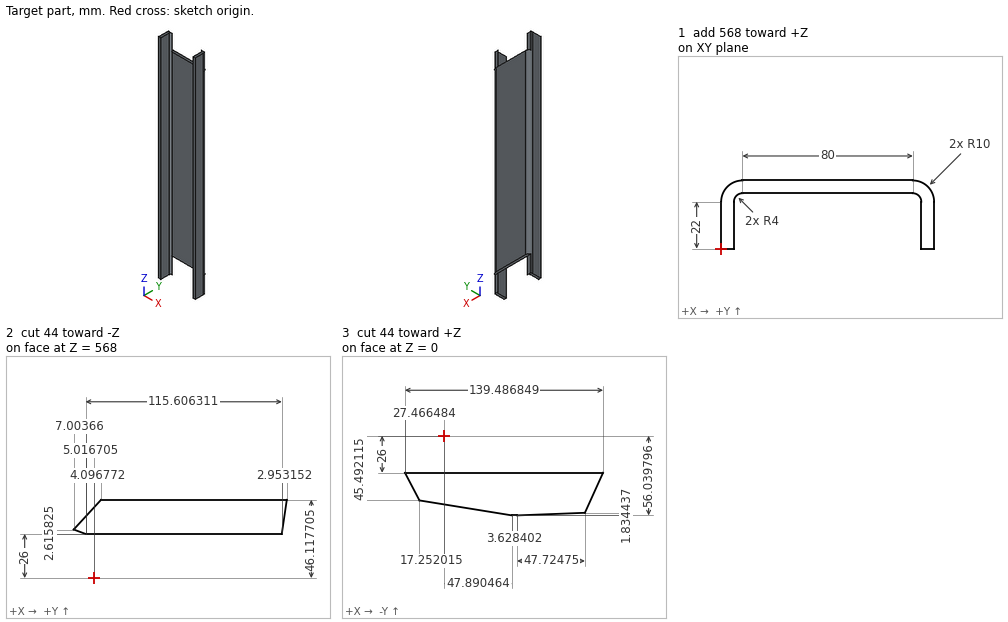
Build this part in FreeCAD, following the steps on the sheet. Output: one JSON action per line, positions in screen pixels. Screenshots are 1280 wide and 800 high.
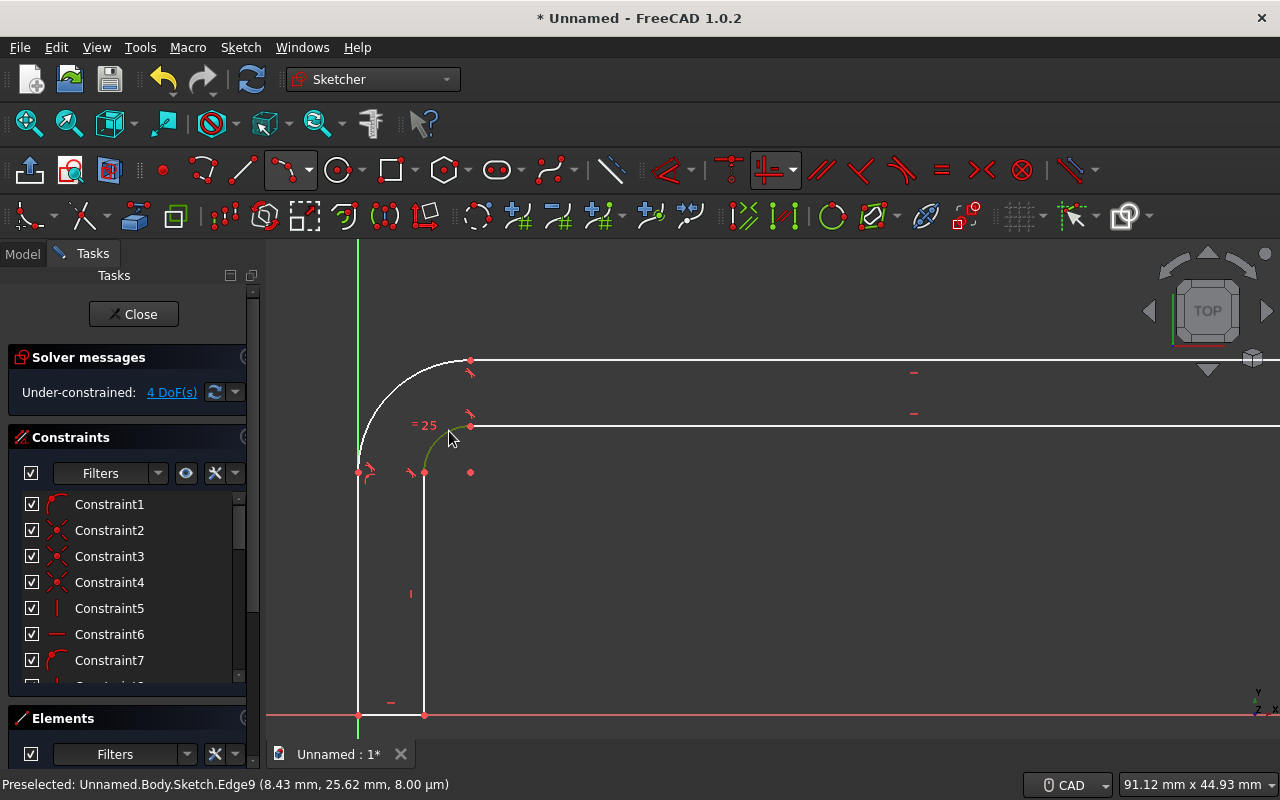
{"action": "left_click", "coordinate": [694, 170]}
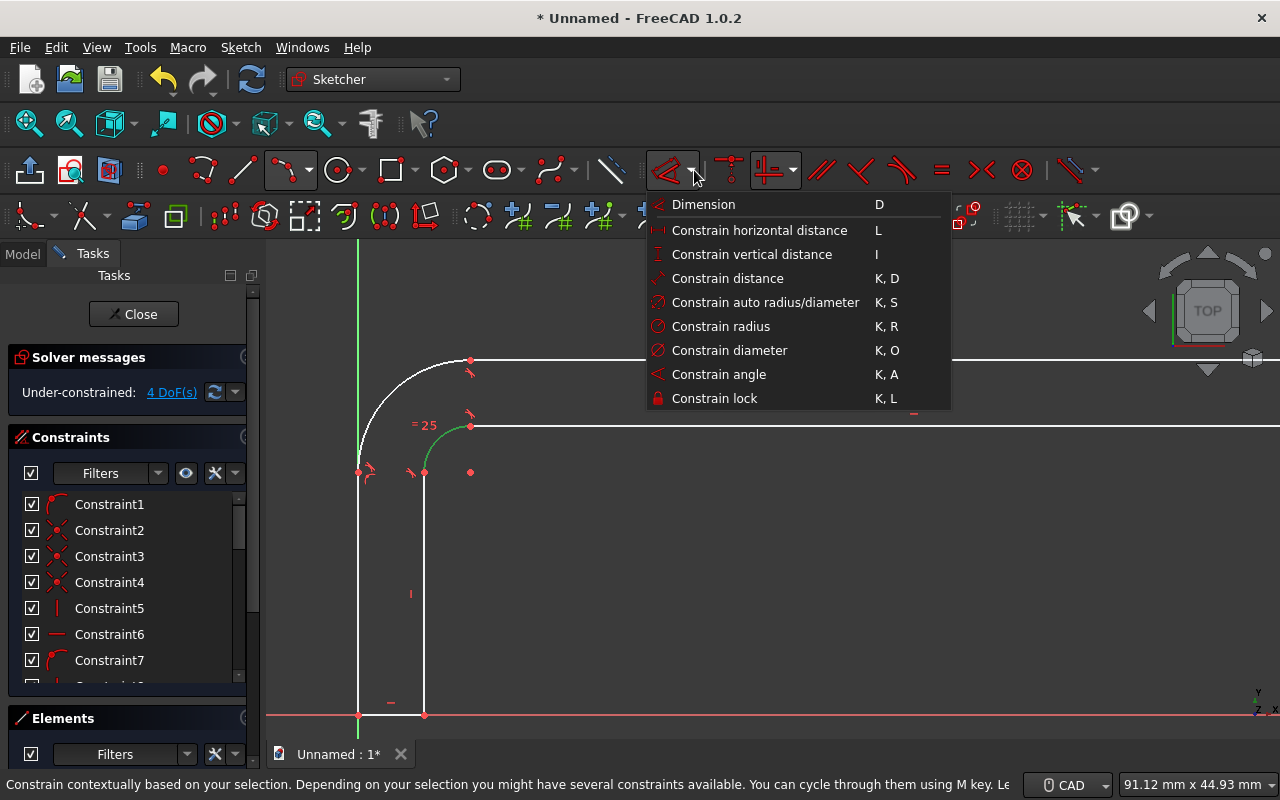
{"action": "left_click", "coordinate": [799, 326]}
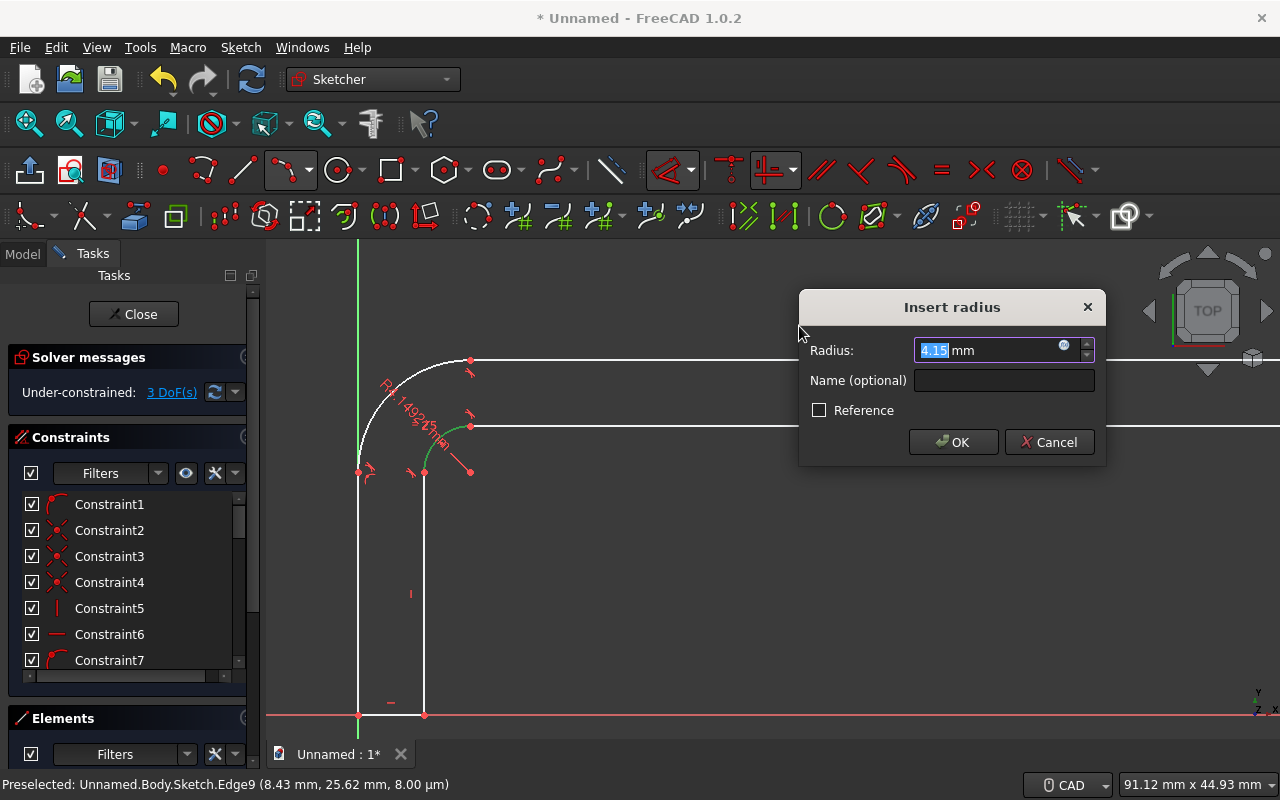
{"action": "type", "text": "4"}
{"action": "key", "text": "Return"}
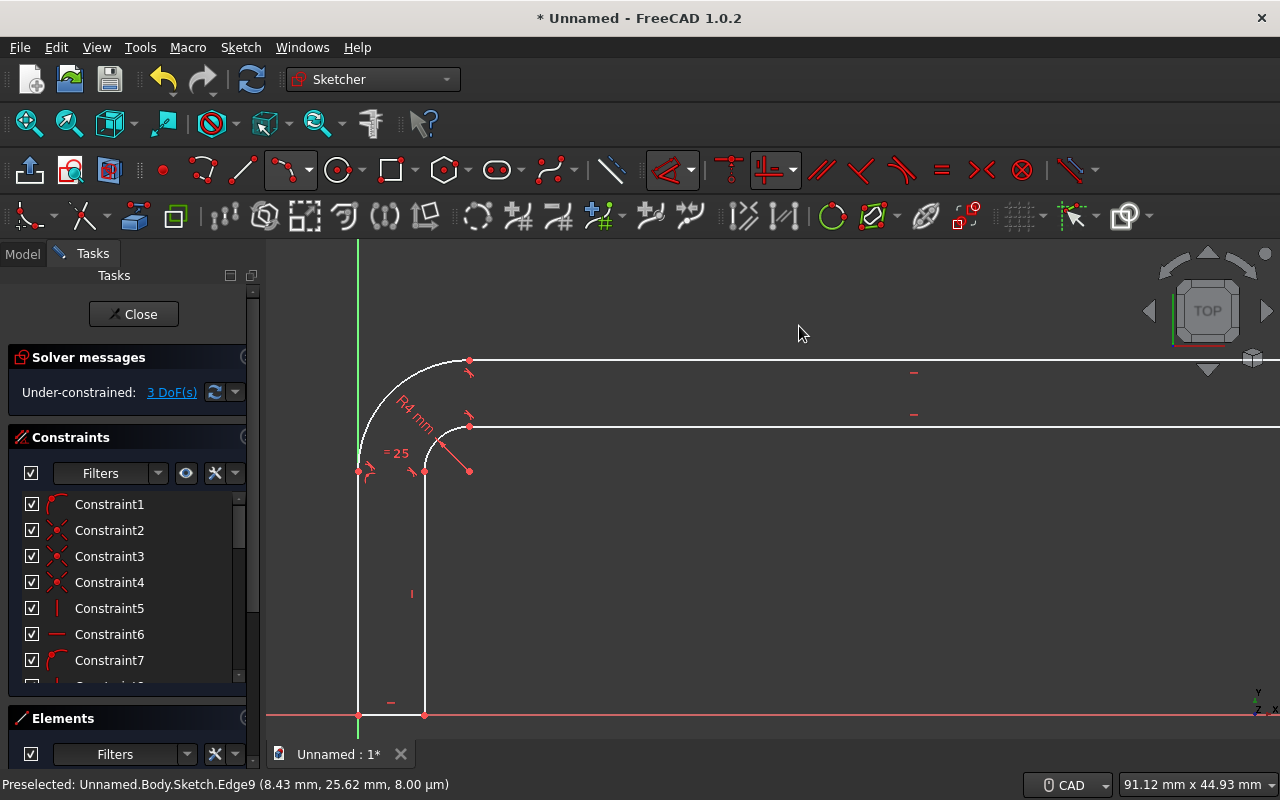
{"action": "scroll", "coordinate": [449, 431], "scroll_direction": "down", "scroll_amount": 3}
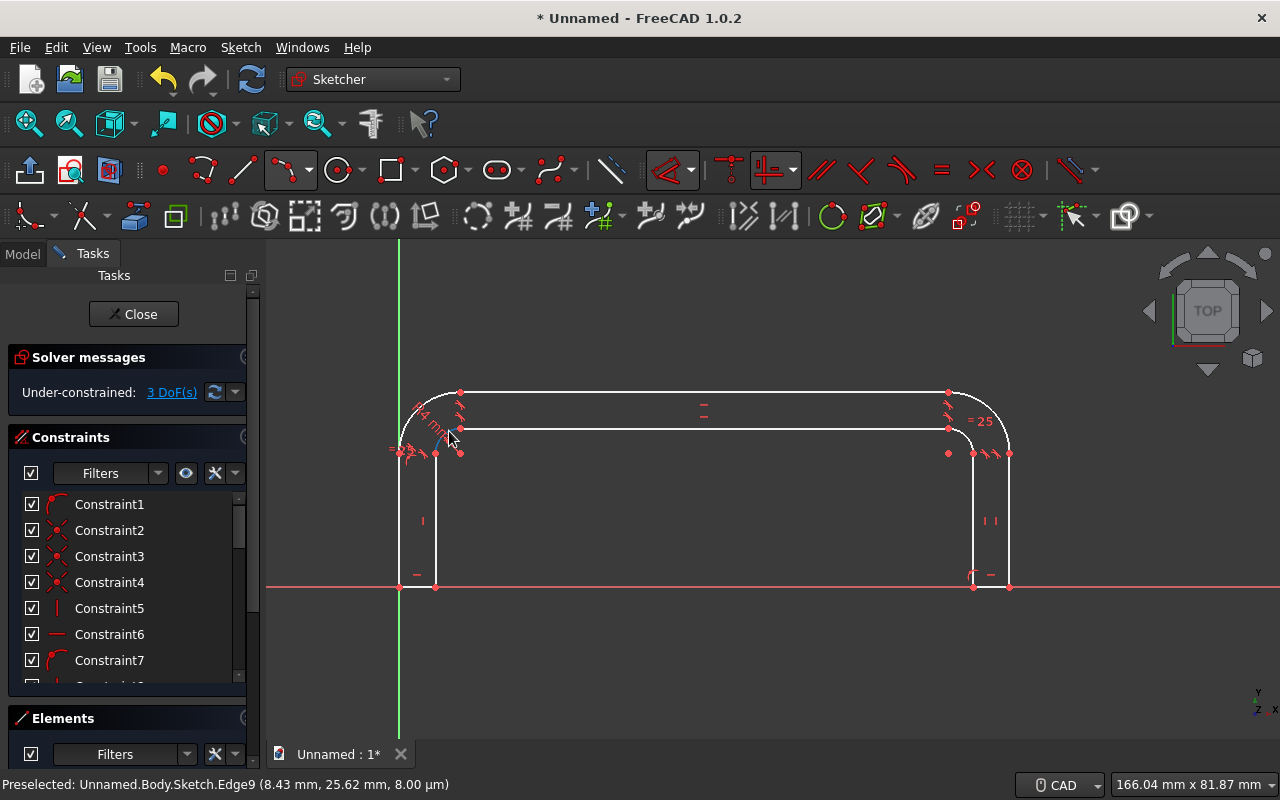
{"action": "left_click", "coordinate": [1003, 426]}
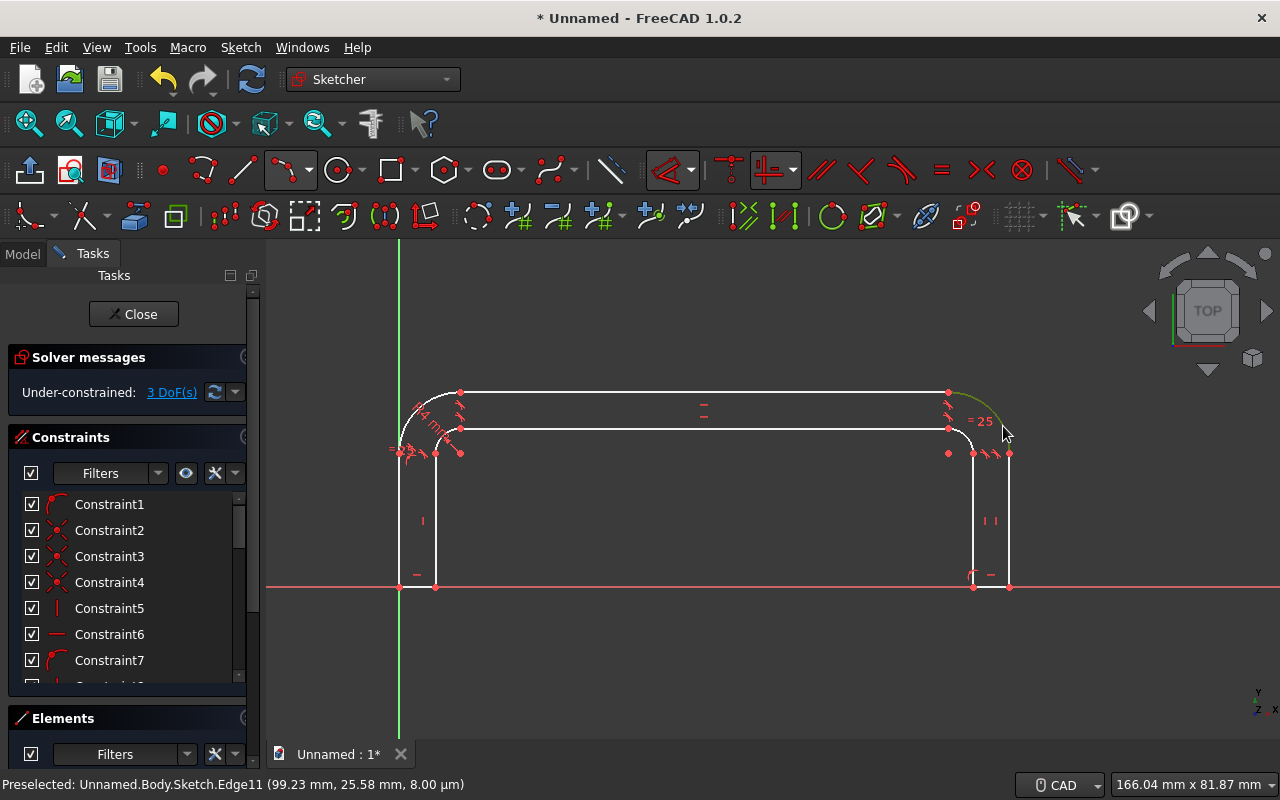
{"action": "key", "text": "k r"}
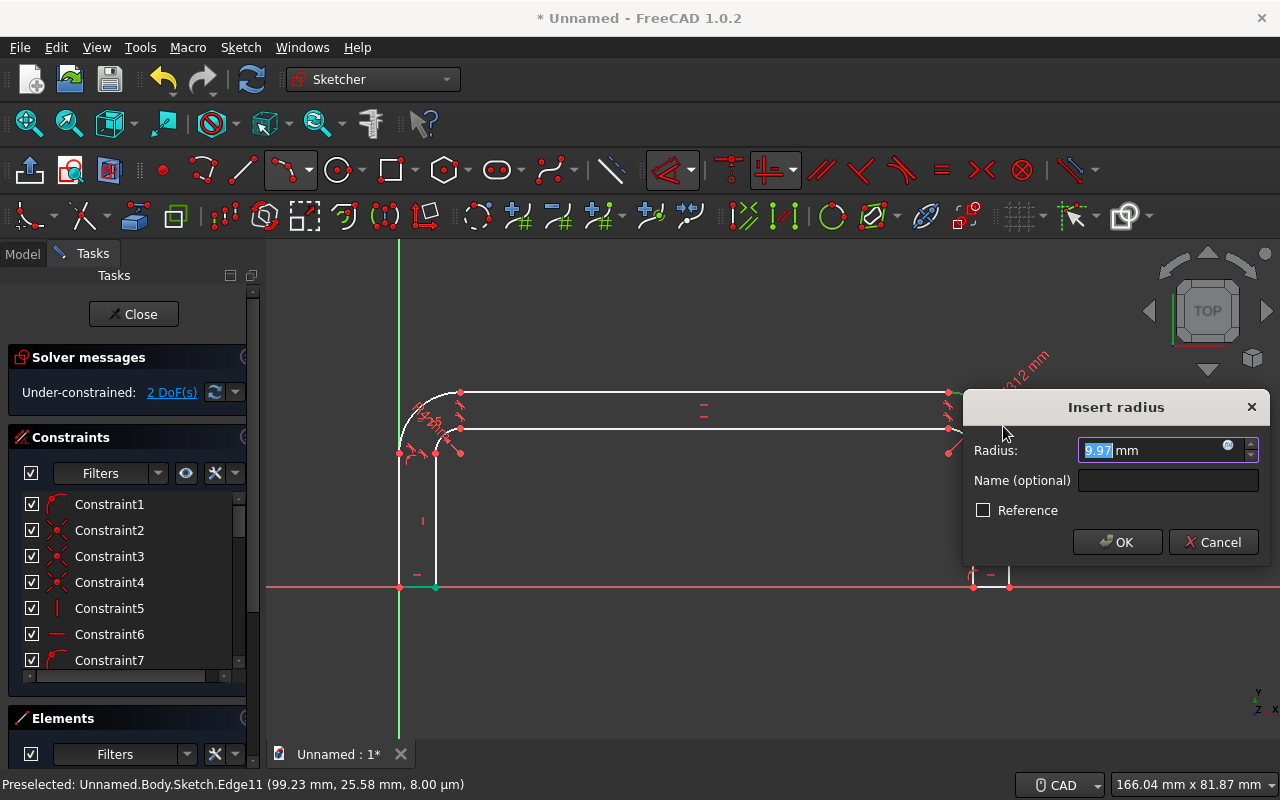
{"action": "type", "text": "10"}
{"action": "key", "text": "Return"}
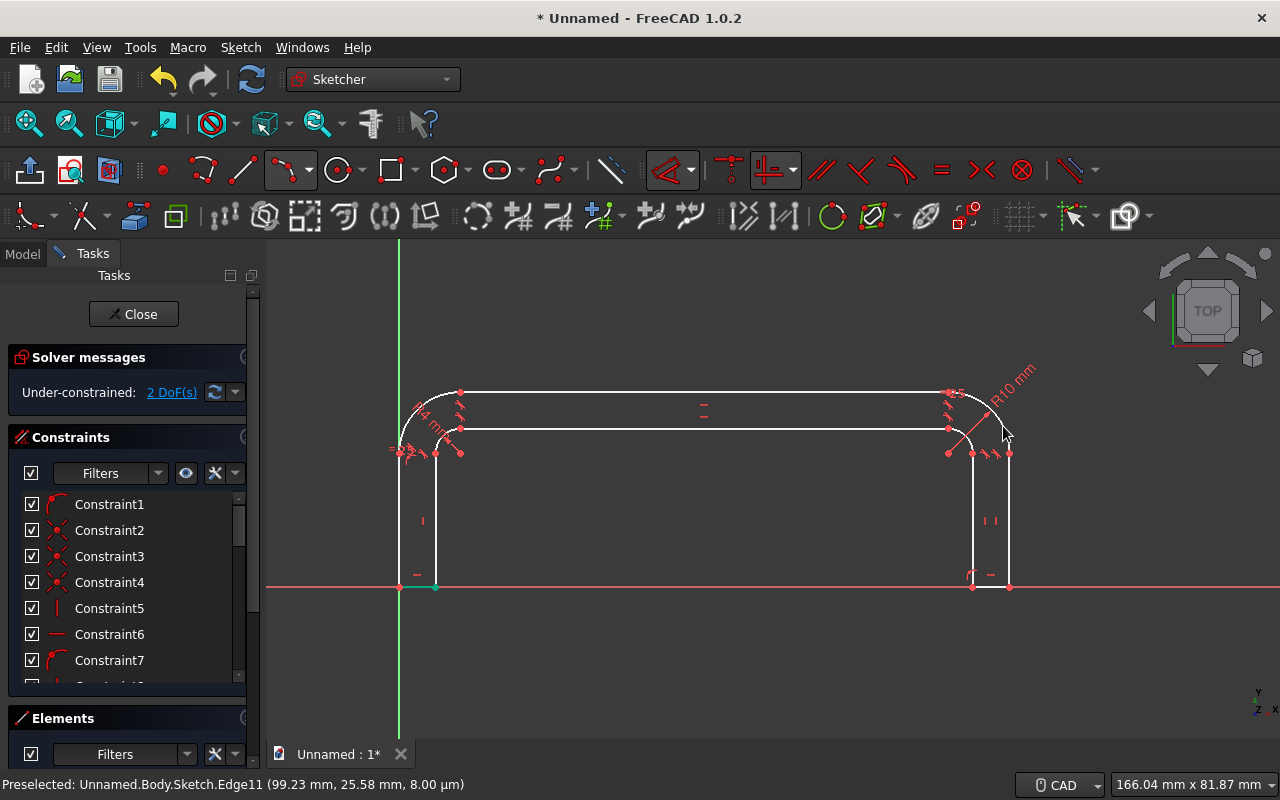
{"action": "left_click", "coordinate": [399, 493]}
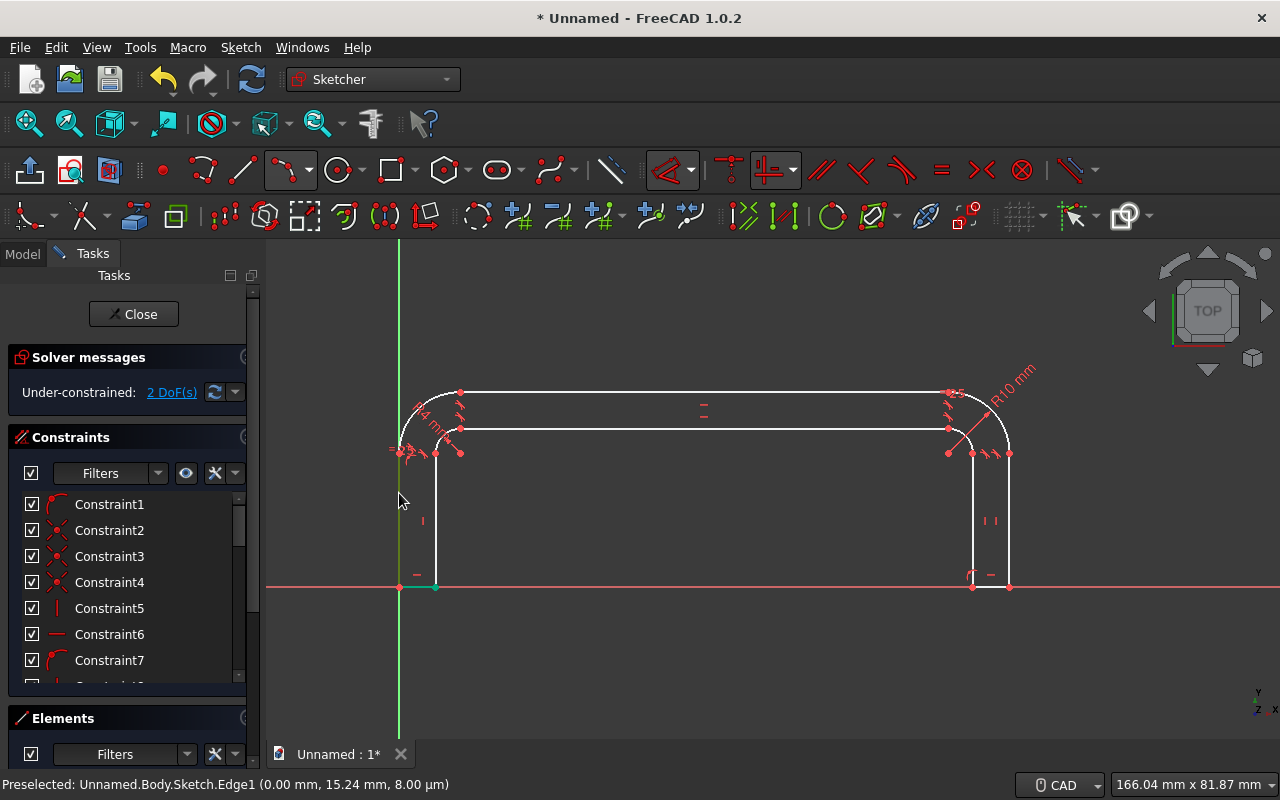
{"action": "left_click", "coordinate": [694, 170]}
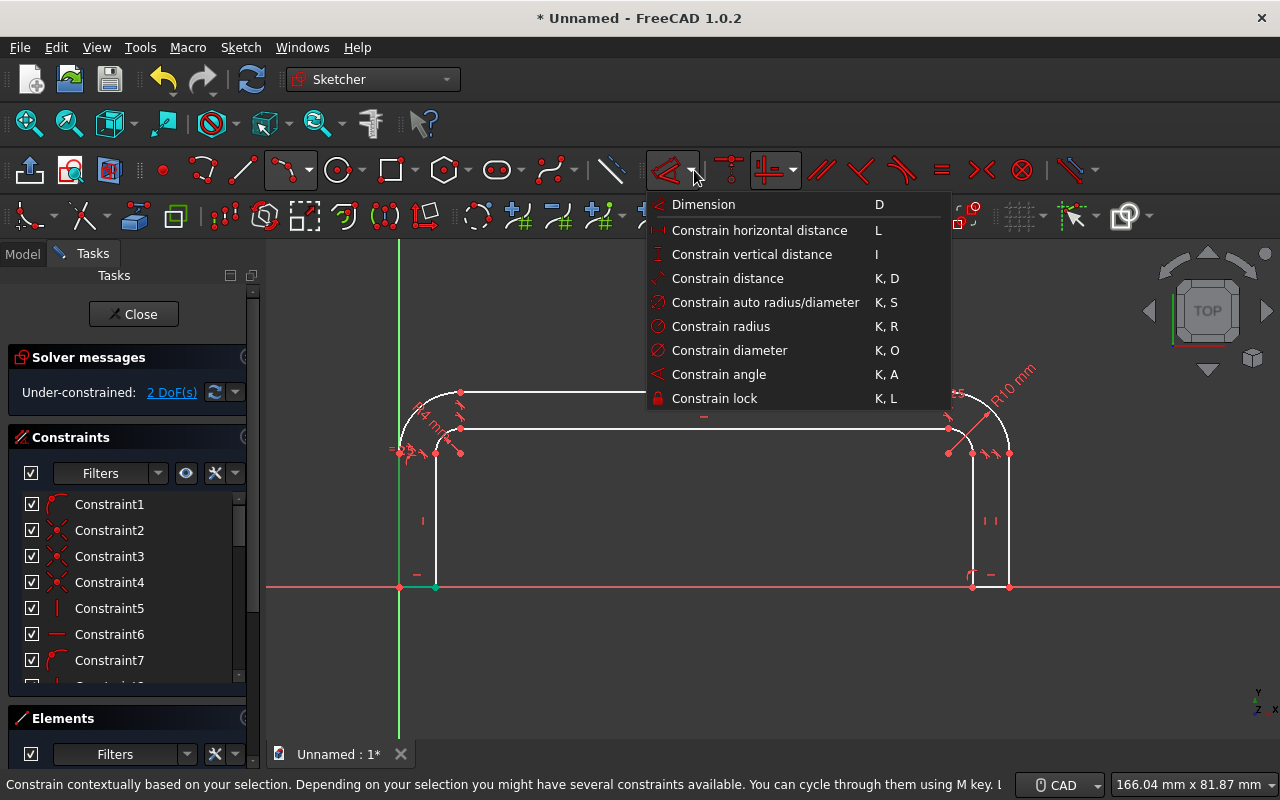
{"action": "left_click", "coordinate": [799, 254]}